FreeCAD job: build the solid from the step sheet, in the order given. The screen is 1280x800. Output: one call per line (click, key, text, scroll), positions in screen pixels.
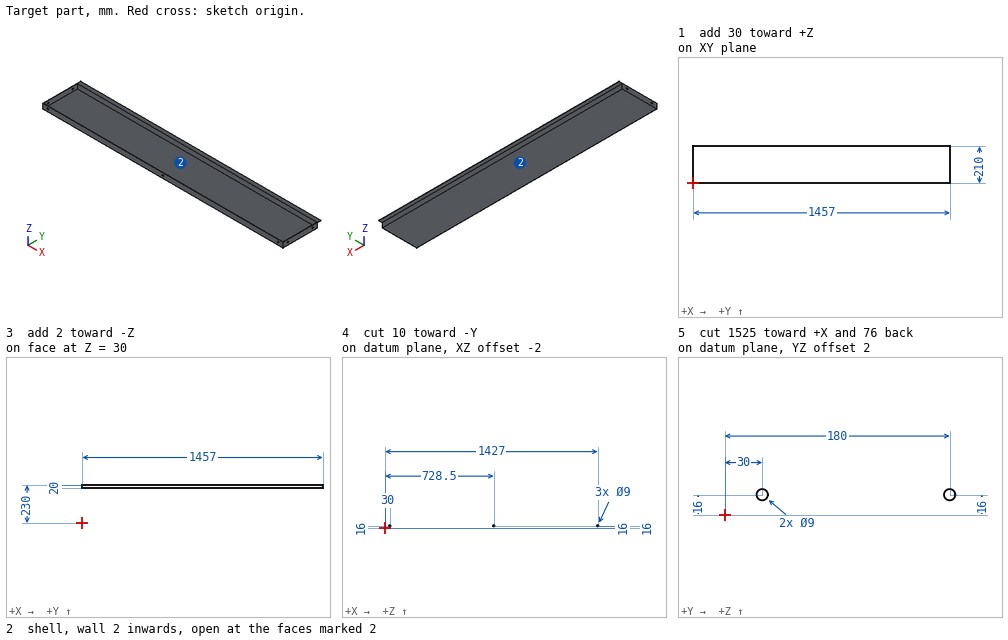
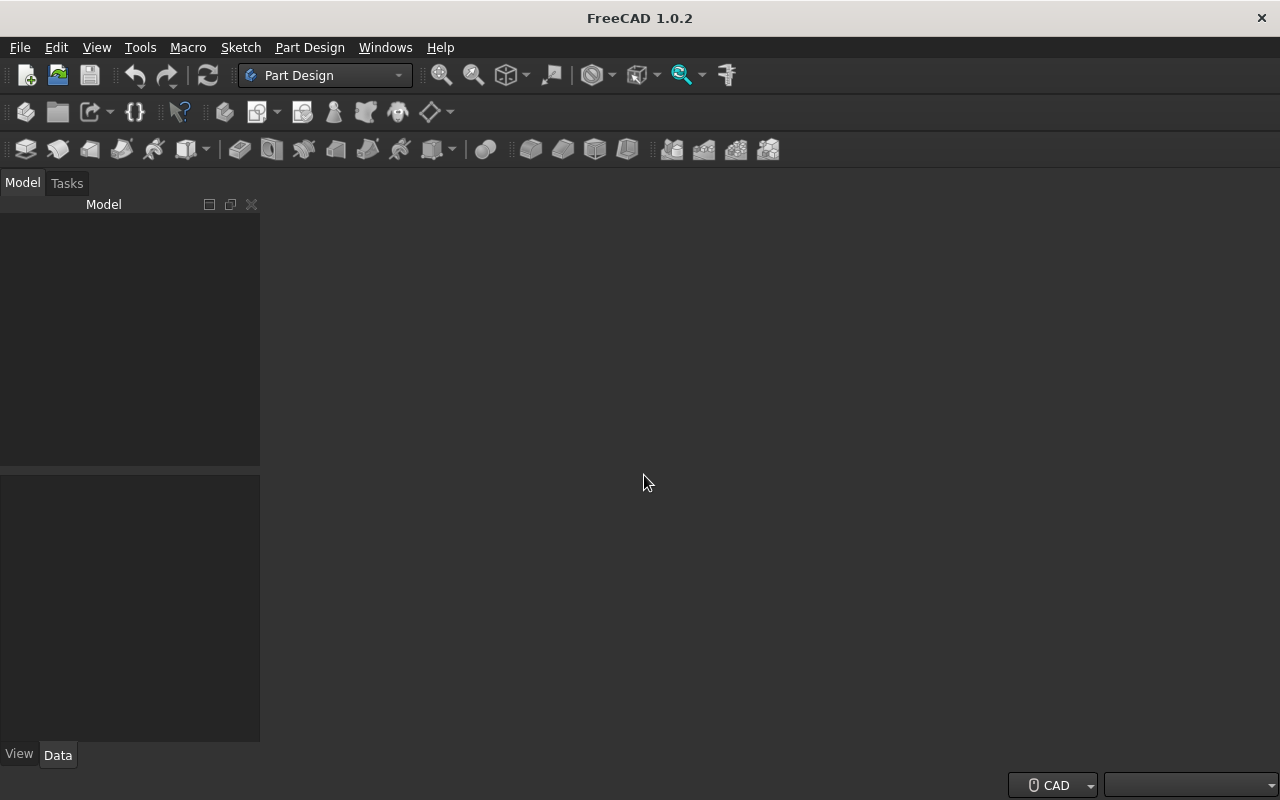
click(26, 76)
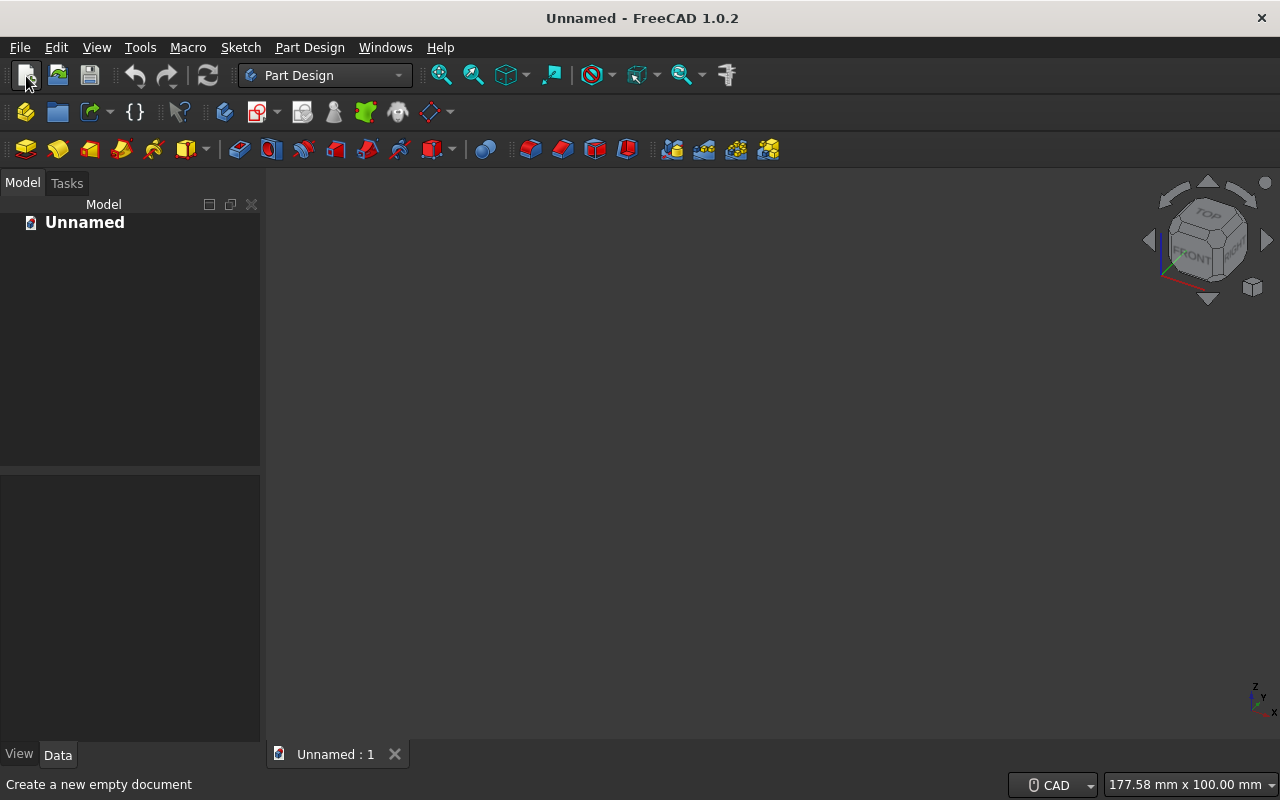
click(258, 112)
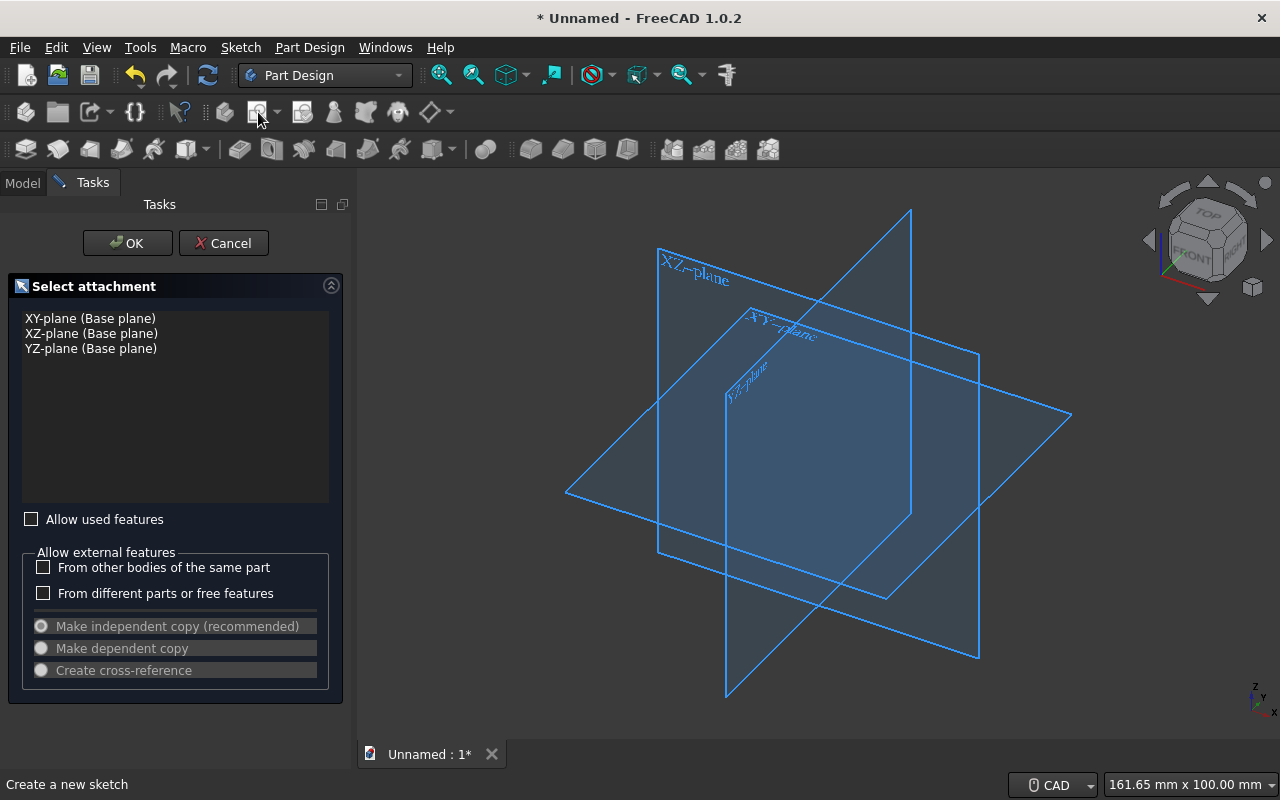
click(82, 318)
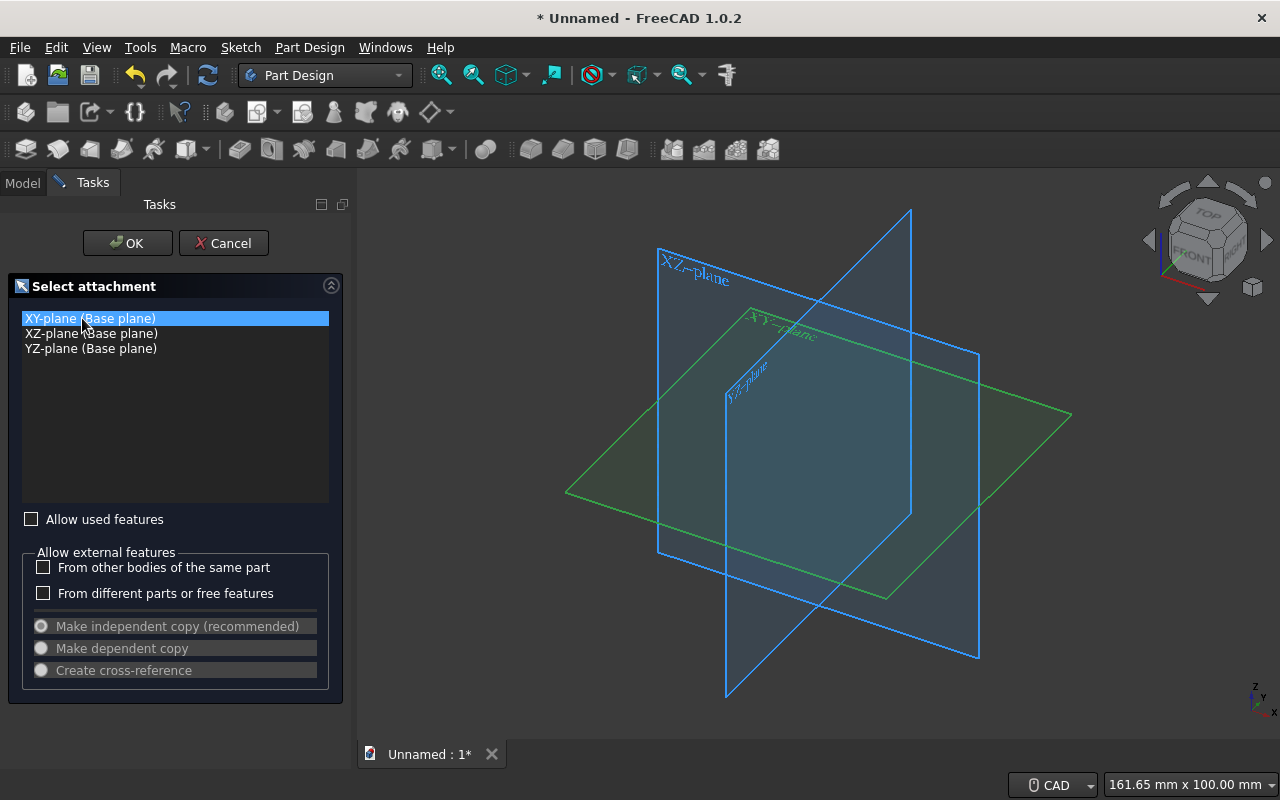
click(128, 243)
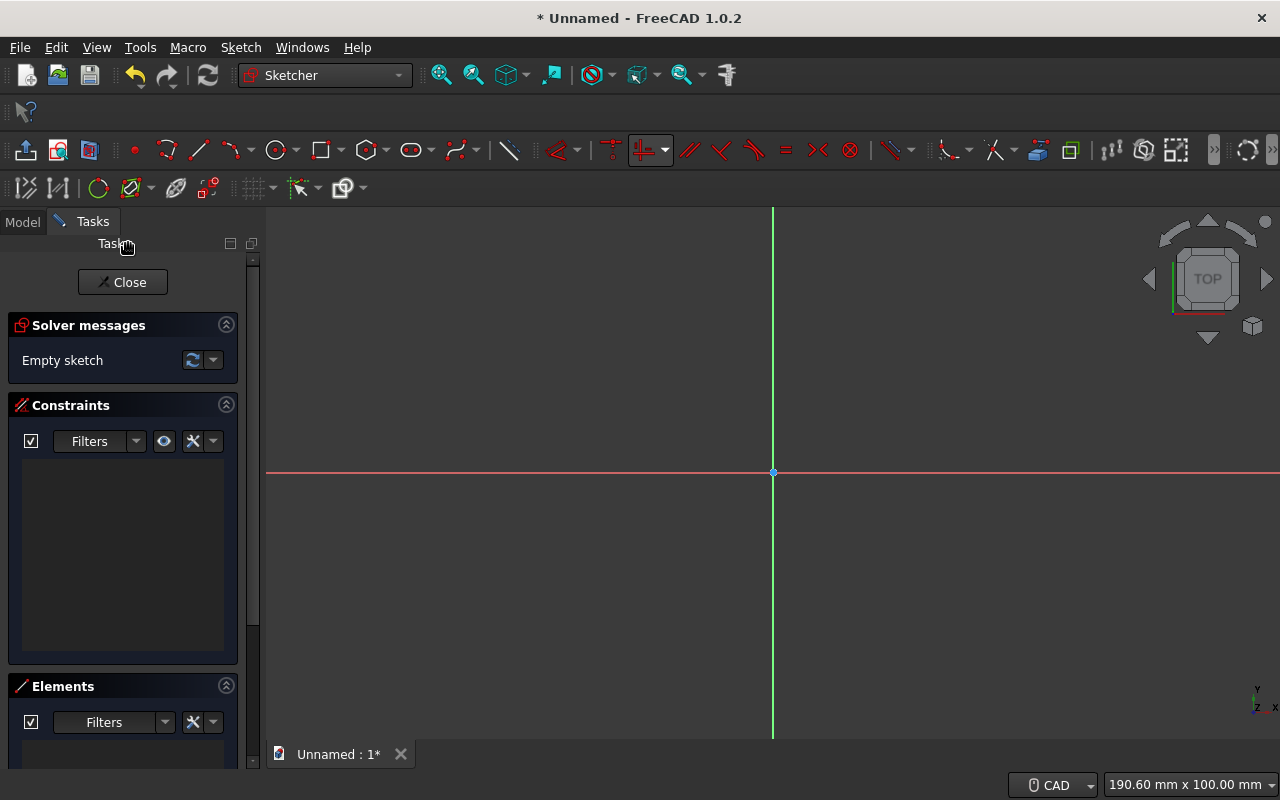
scroll(388, 518, down, 13)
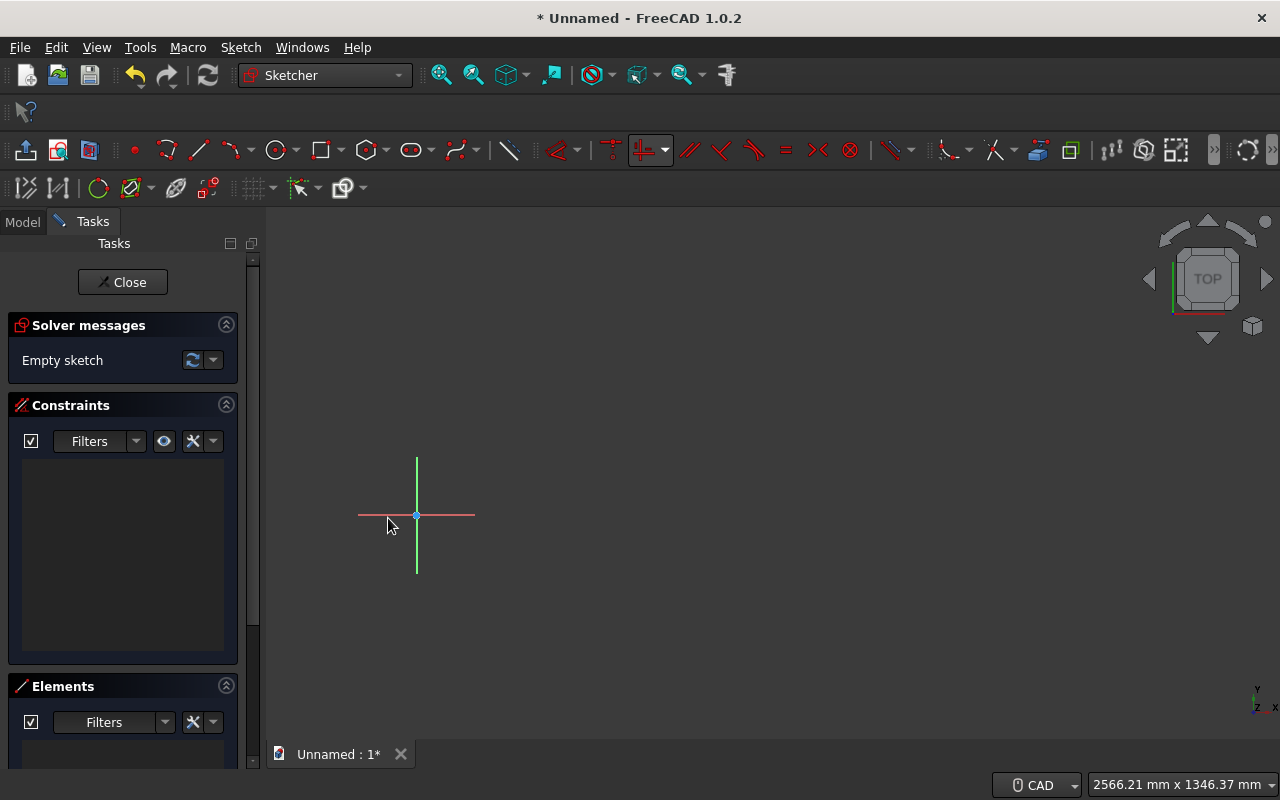
click(322, 150)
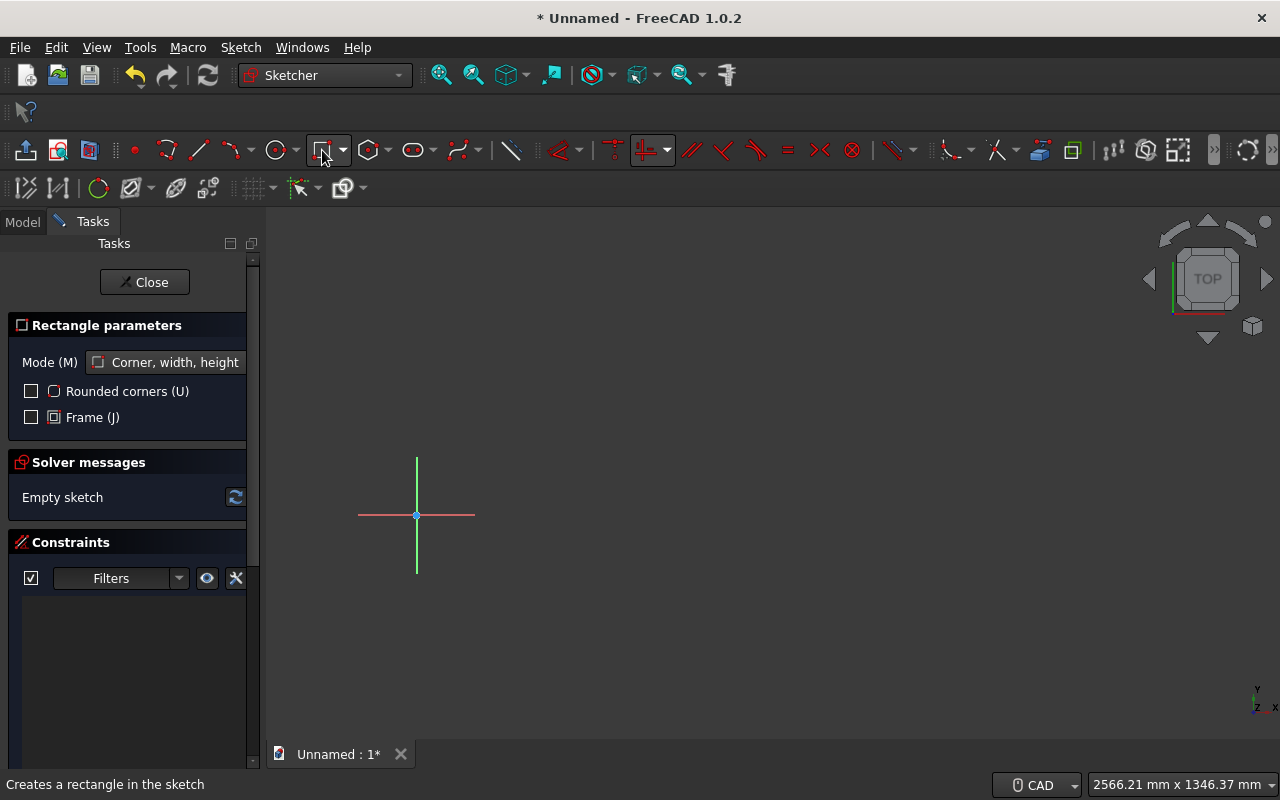
click(417, 515)
move(992, 432)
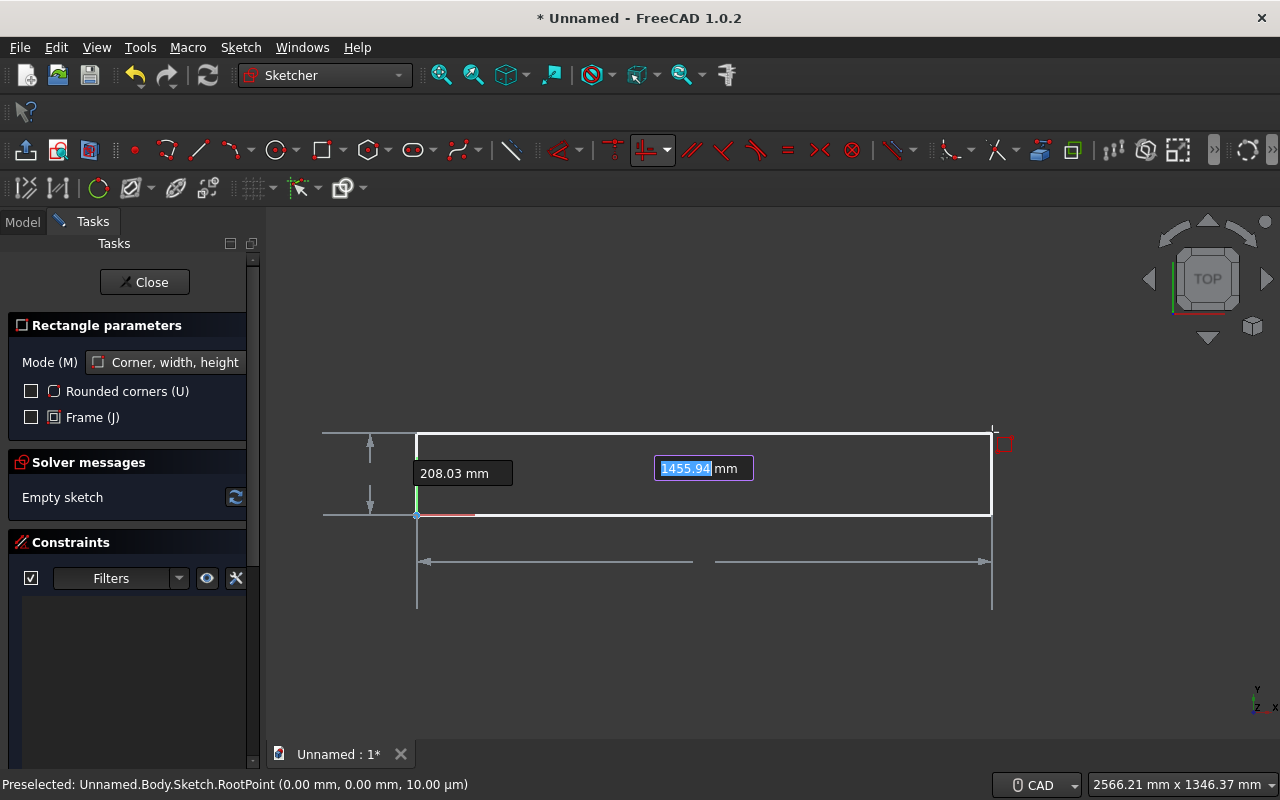
text(1457)
key(Tab)
text(210)
key(Return)
key(Escape)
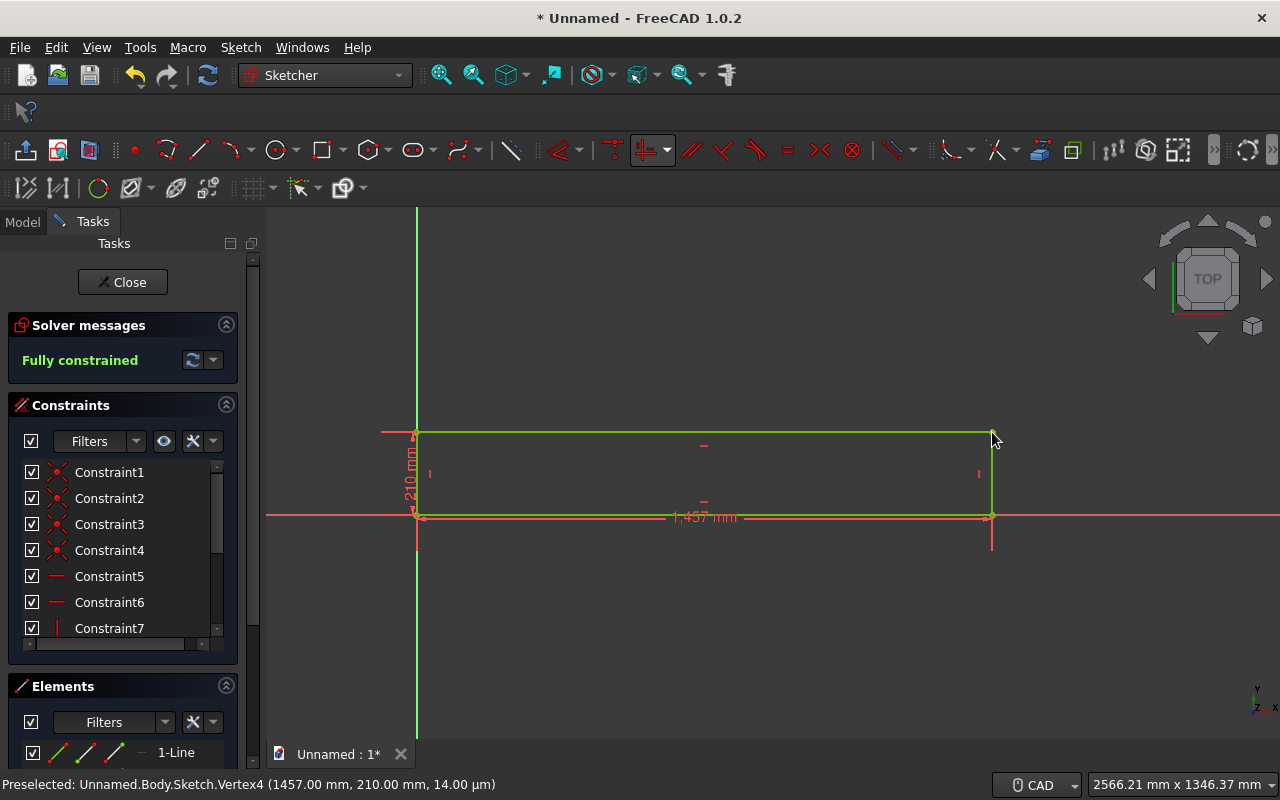
click(123, 282)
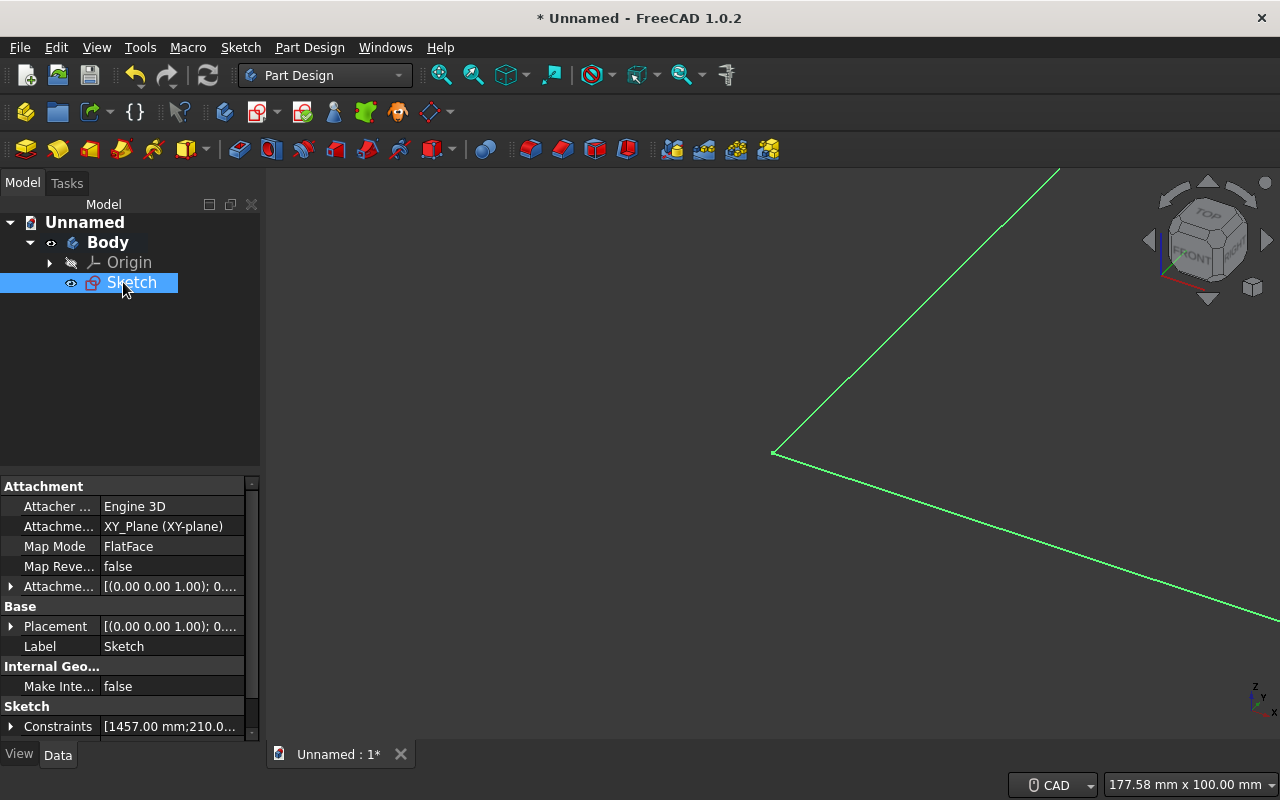
click(26, 150)